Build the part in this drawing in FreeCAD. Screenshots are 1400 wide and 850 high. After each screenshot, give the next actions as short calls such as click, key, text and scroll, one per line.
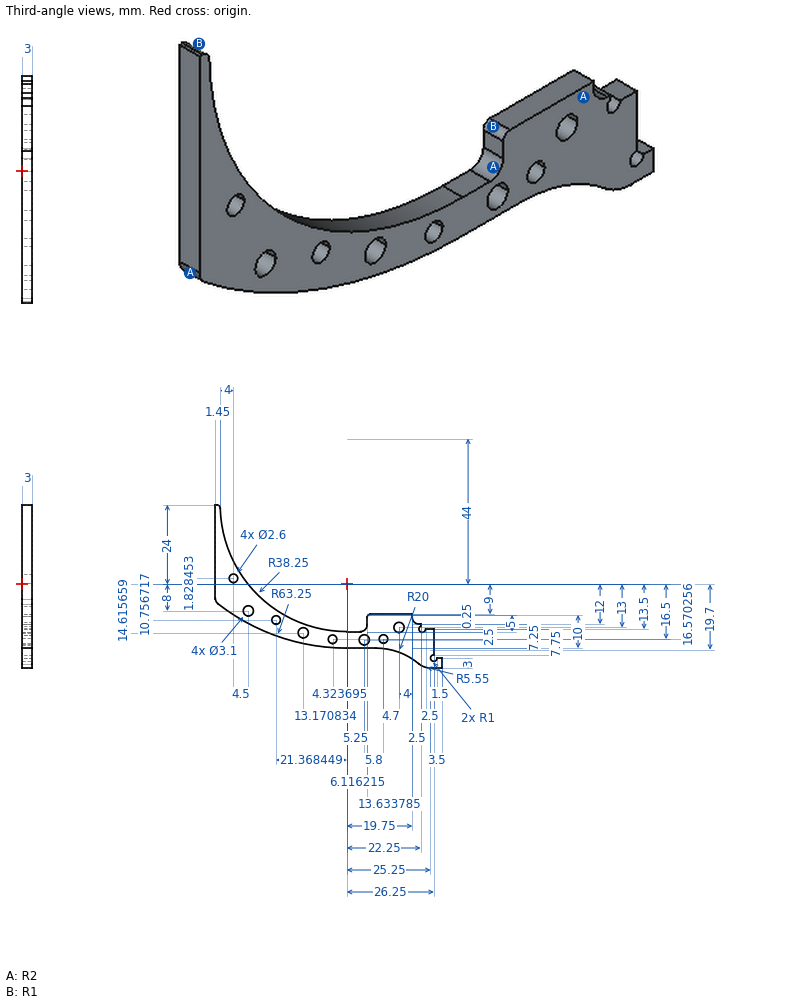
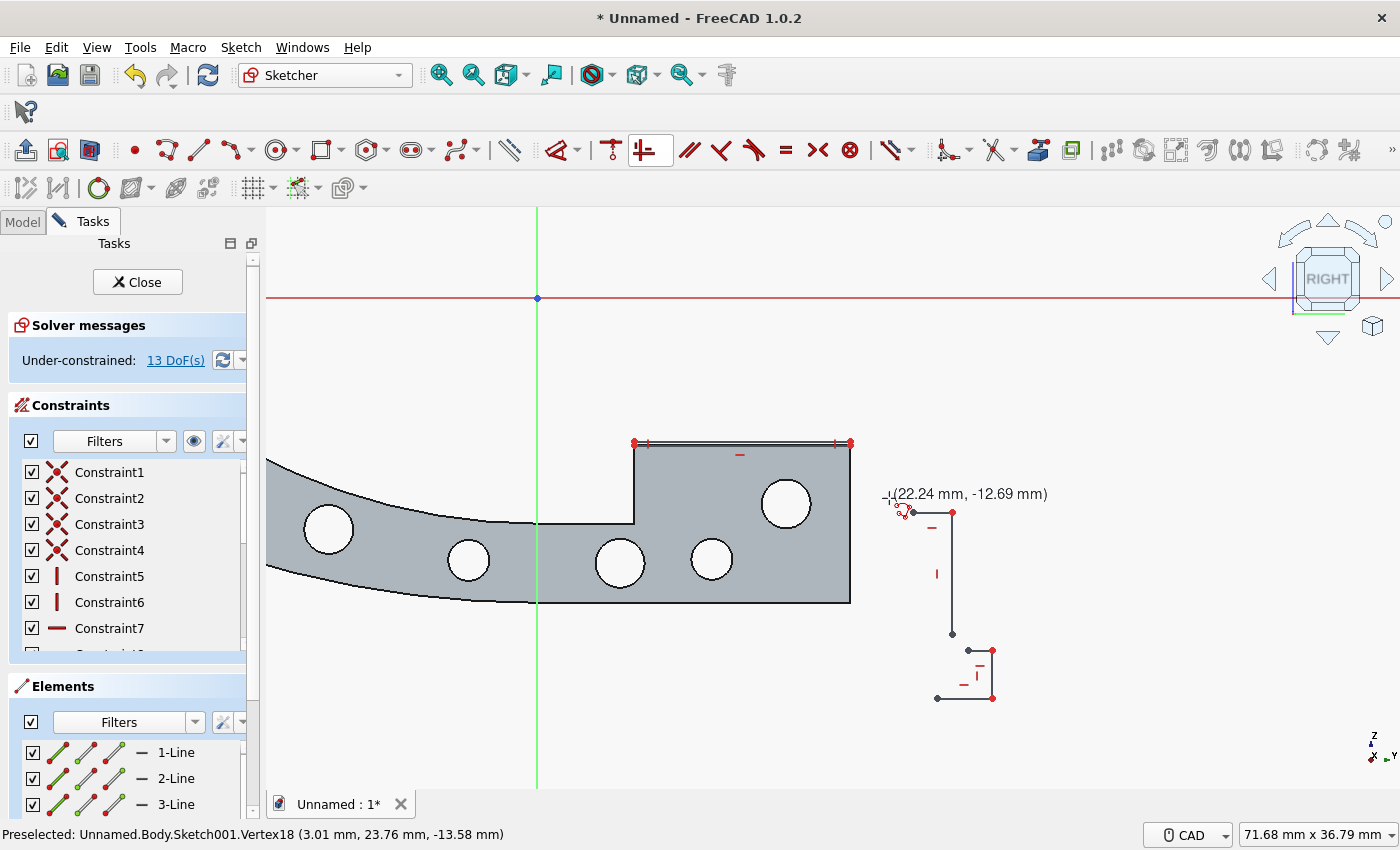
scroll(889, 488, up, 3)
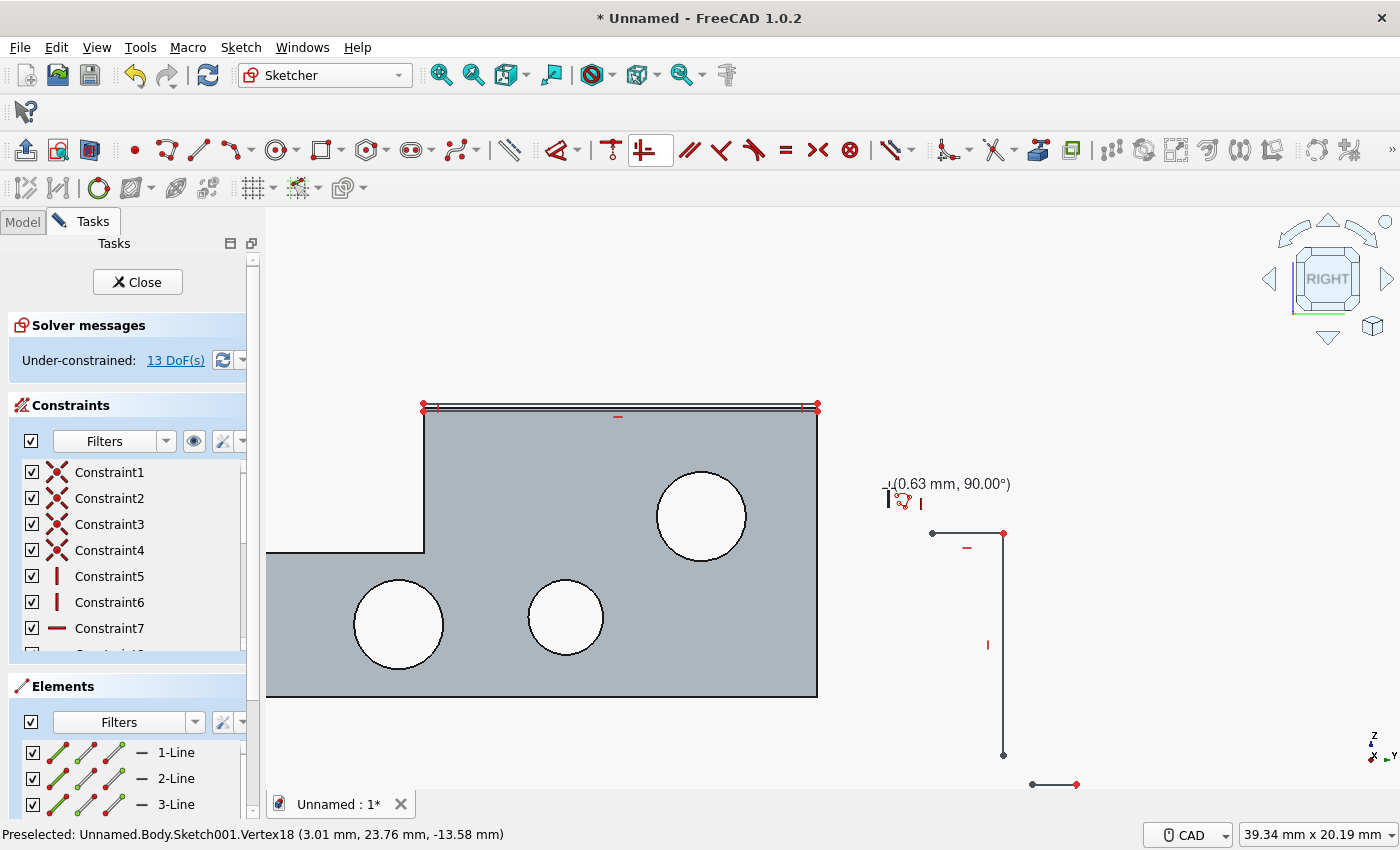
click(889, 488)
click(817, 488)
click(817, 697)
click(501, 697)
right_click(501, 697)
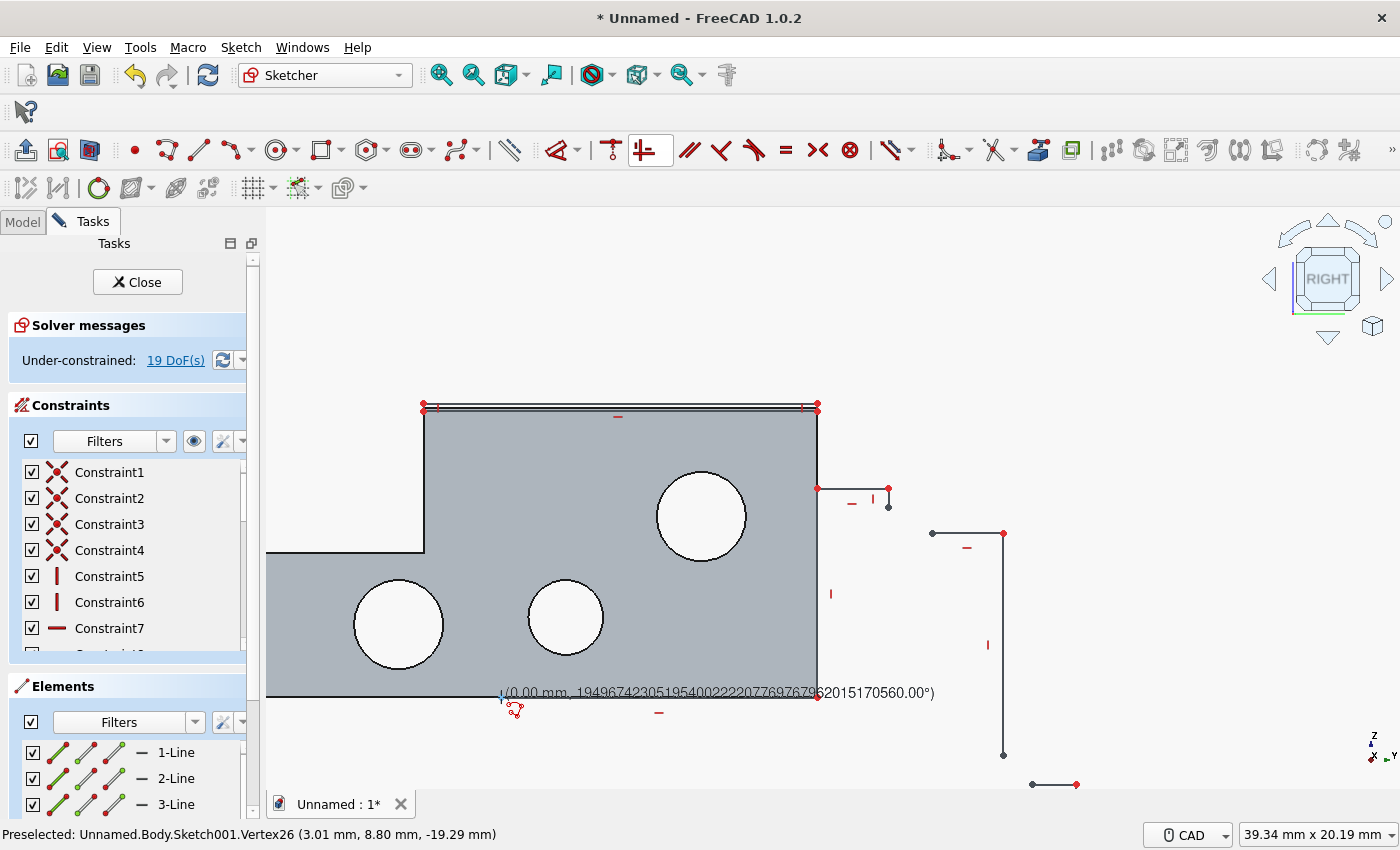
click(232, 150)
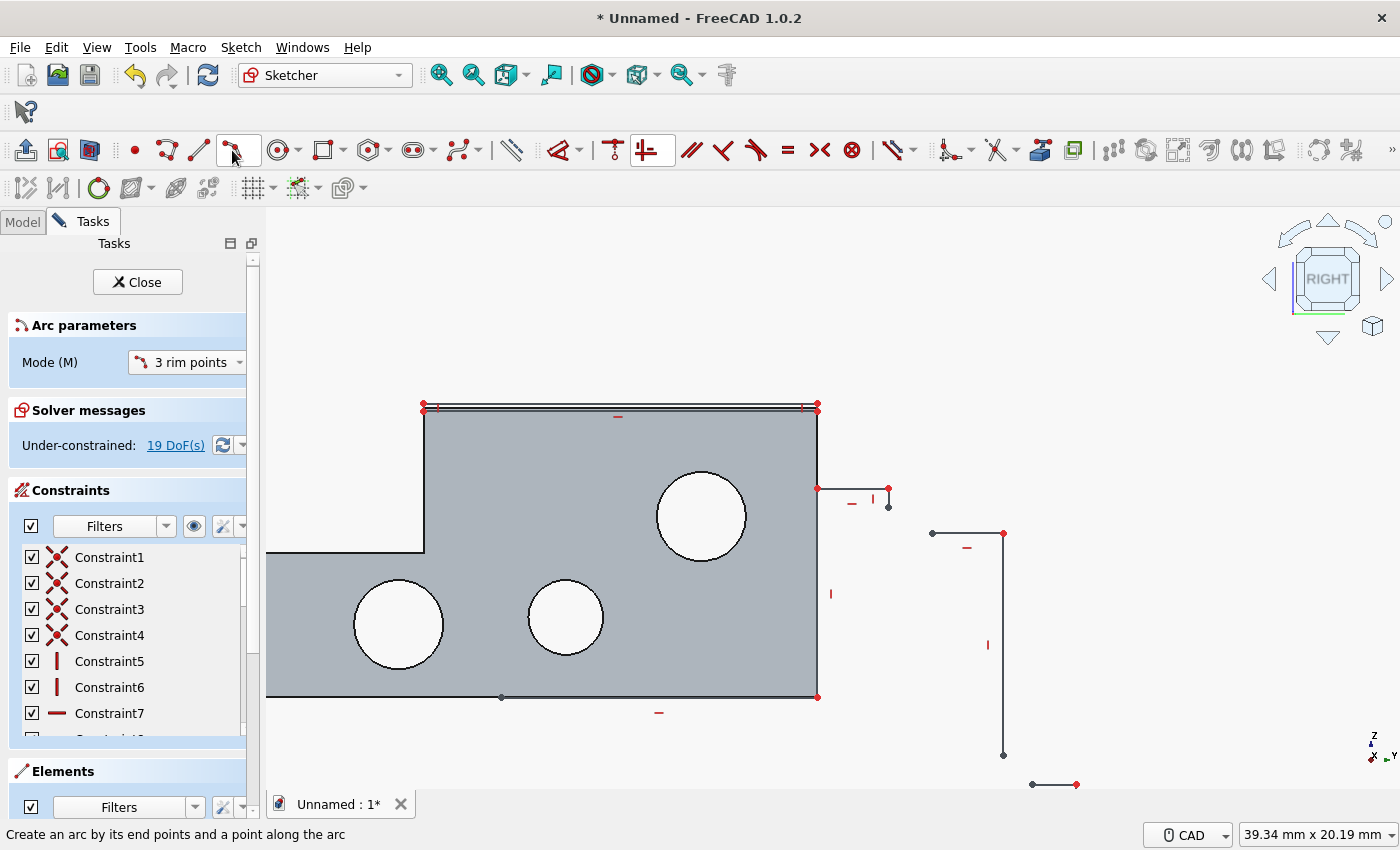
scroll(890, 489, down, 3)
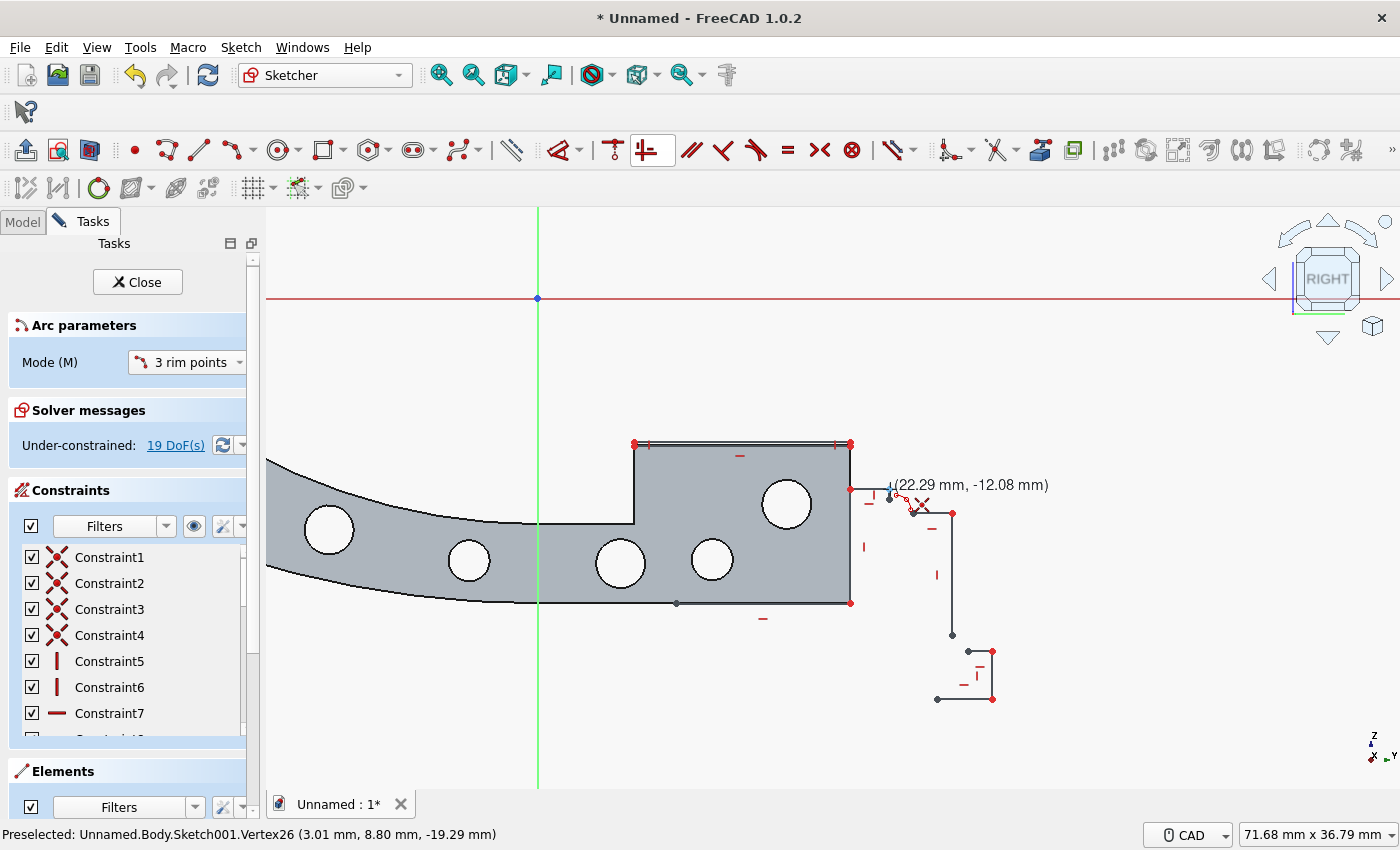
scroll(969, 651, up, 2)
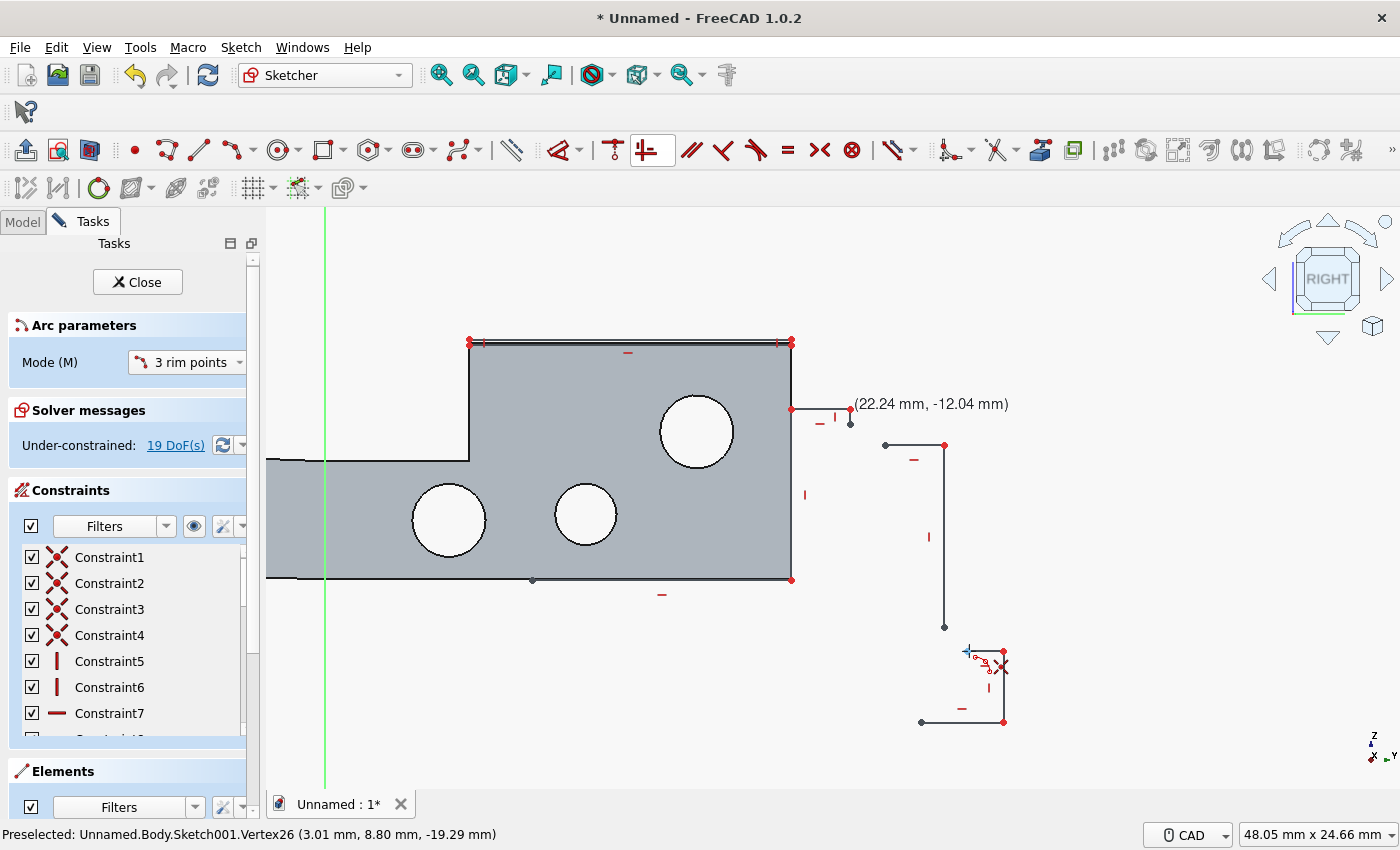
click(968, 651)
click(944, 627)
click(928, 667)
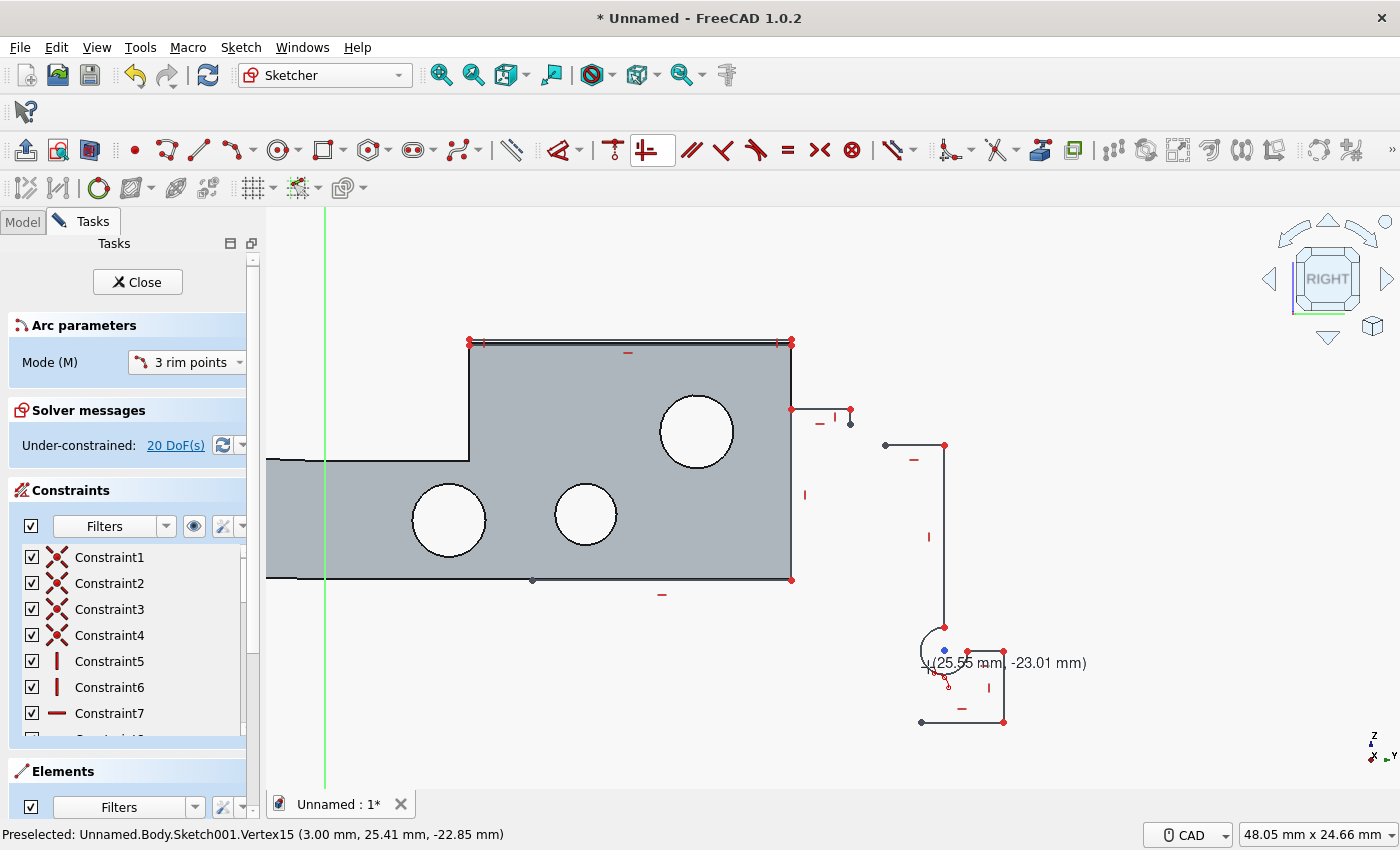
click(886, 445)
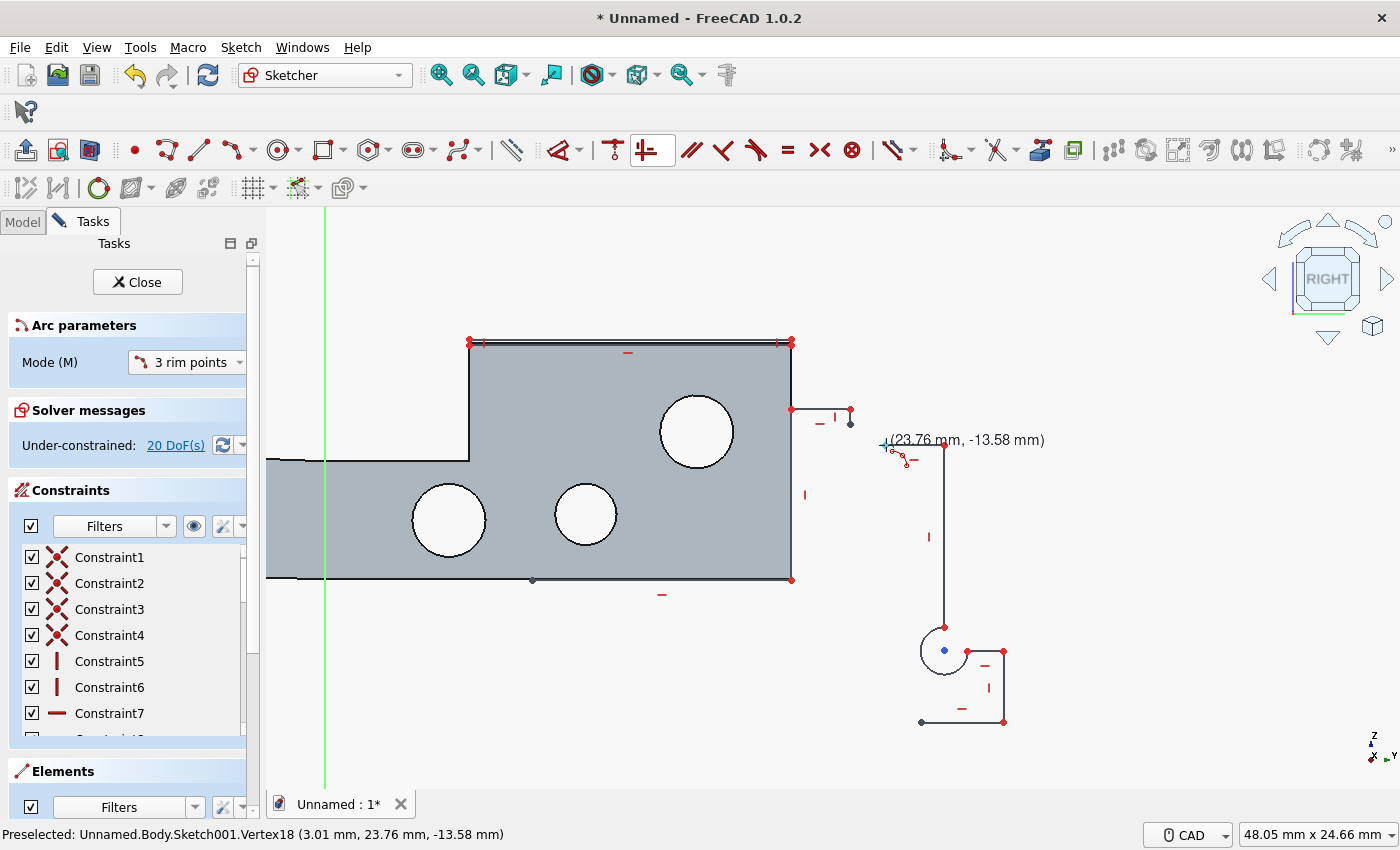
scroll(850, 423, up, 4)